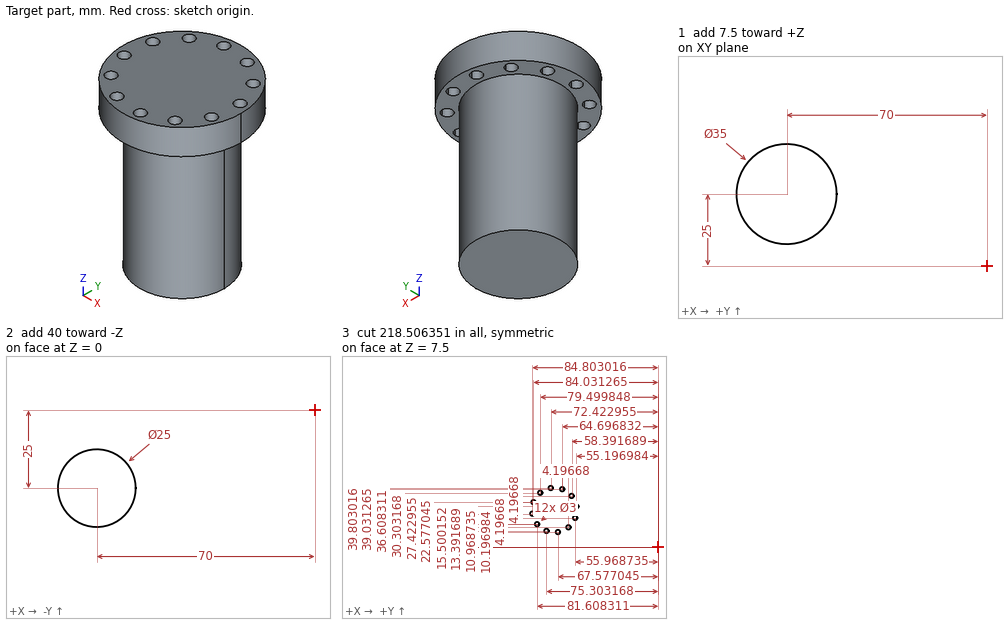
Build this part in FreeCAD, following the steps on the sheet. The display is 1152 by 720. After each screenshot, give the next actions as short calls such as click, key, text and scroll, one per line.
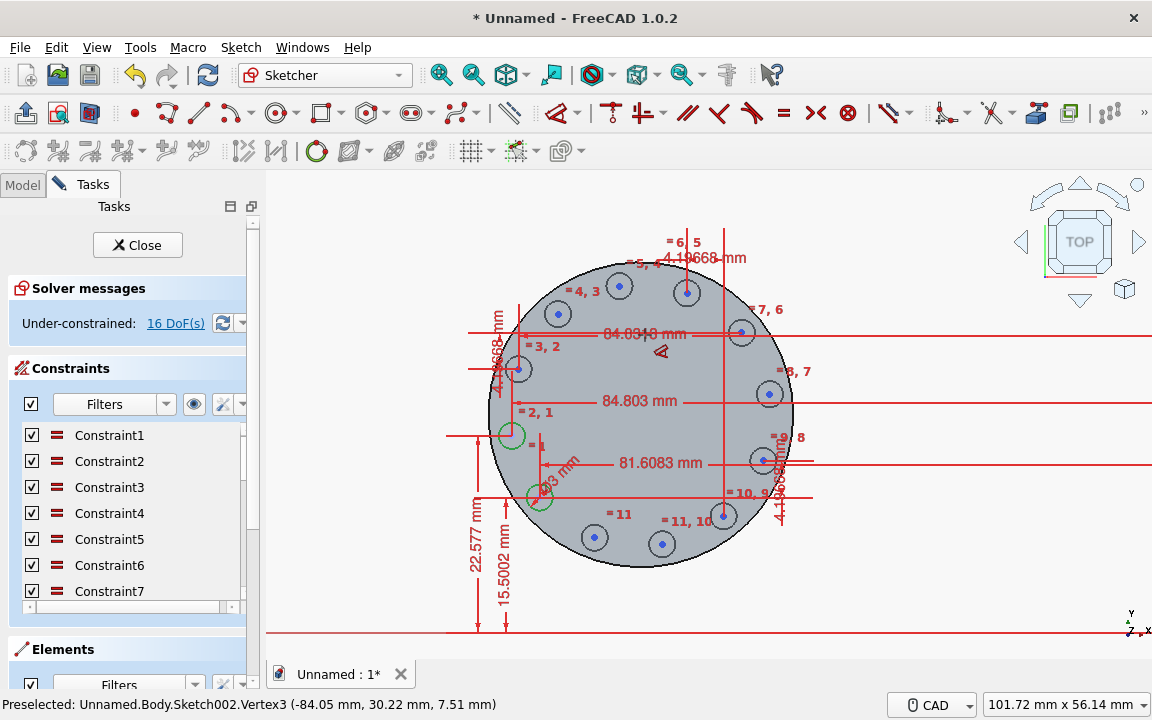
click(519, 369)
click(485, 500)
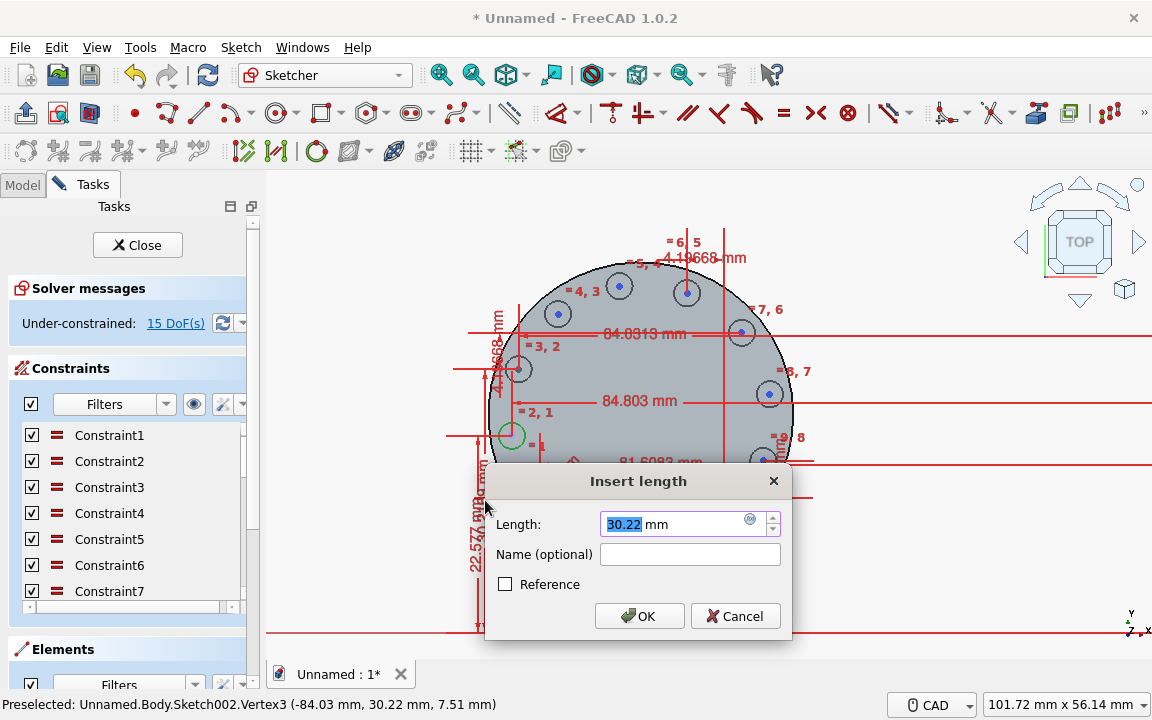
text(30.303168)
key(Return)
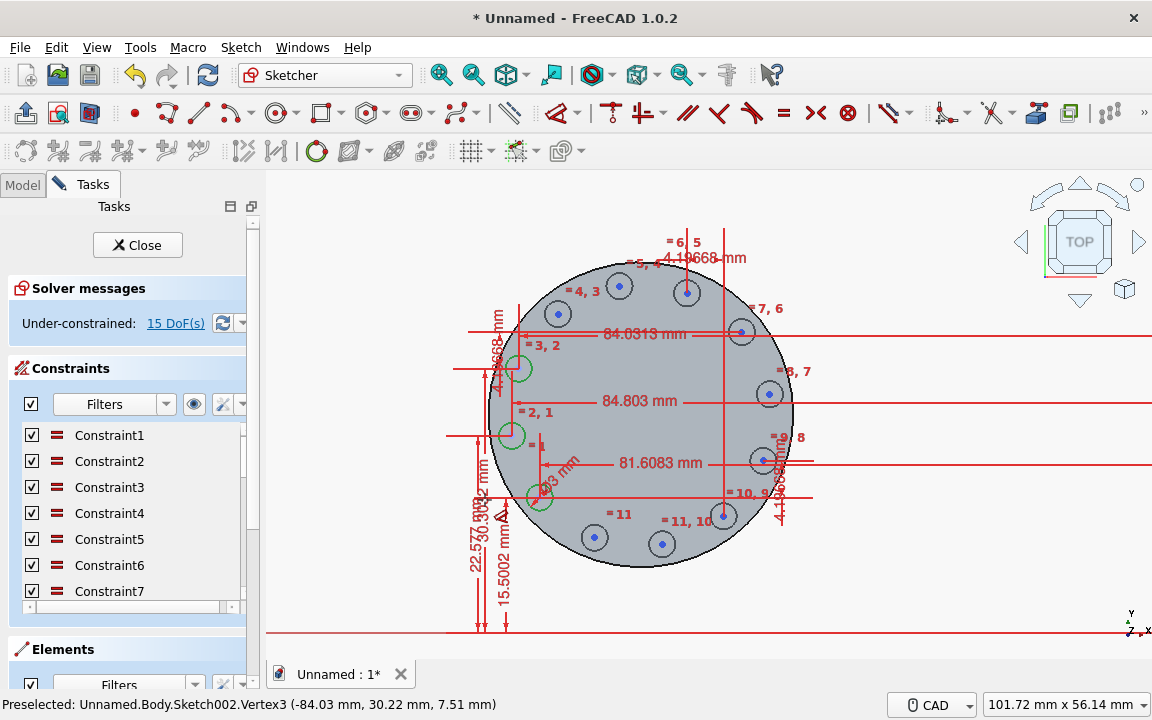
click(558, 314)
click(773, 280)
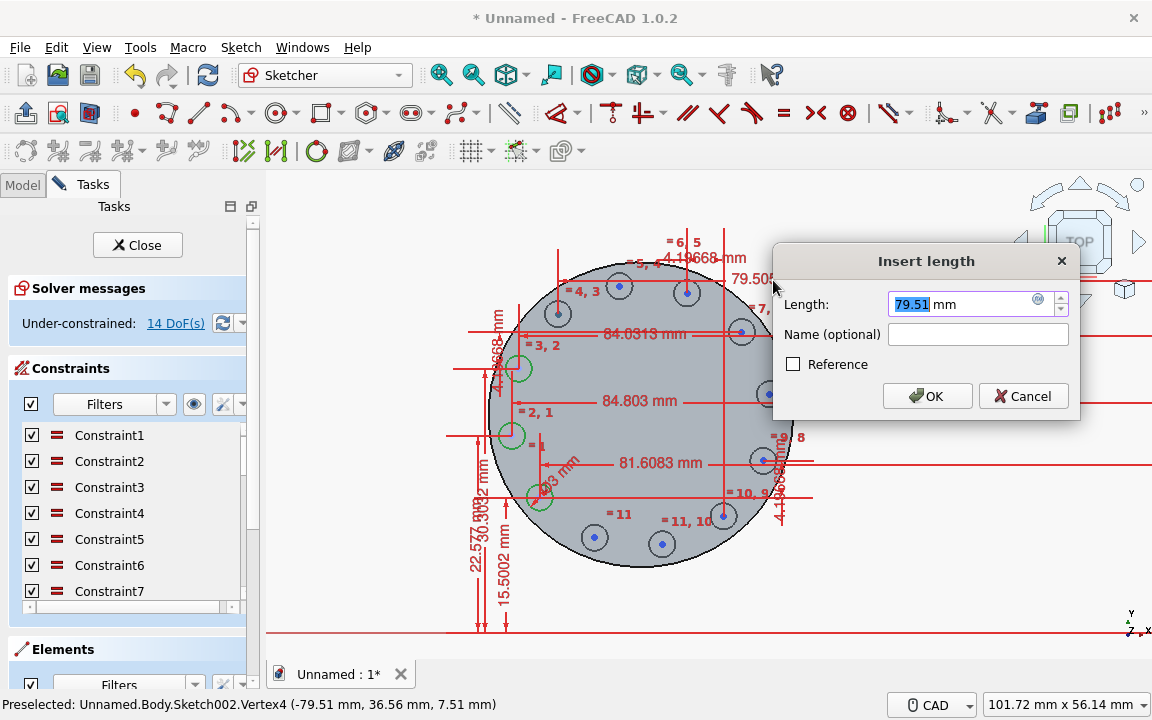
text(79.499848)
key(Return)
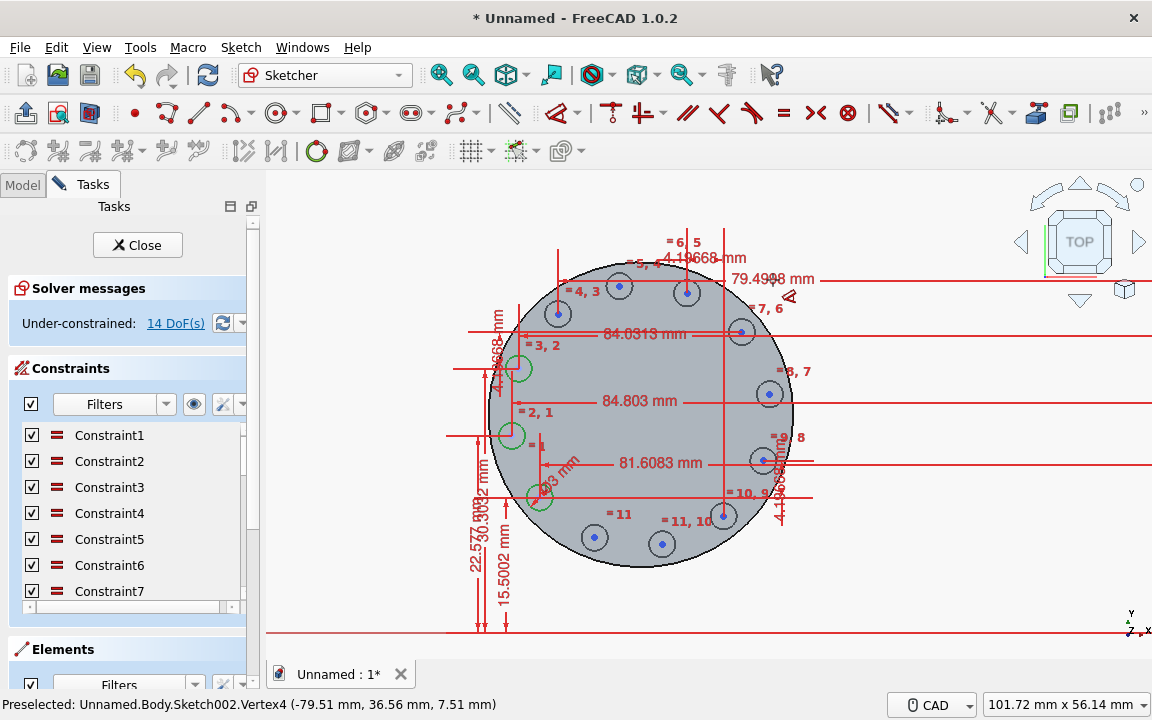
click(558, 314)
click(524, 400)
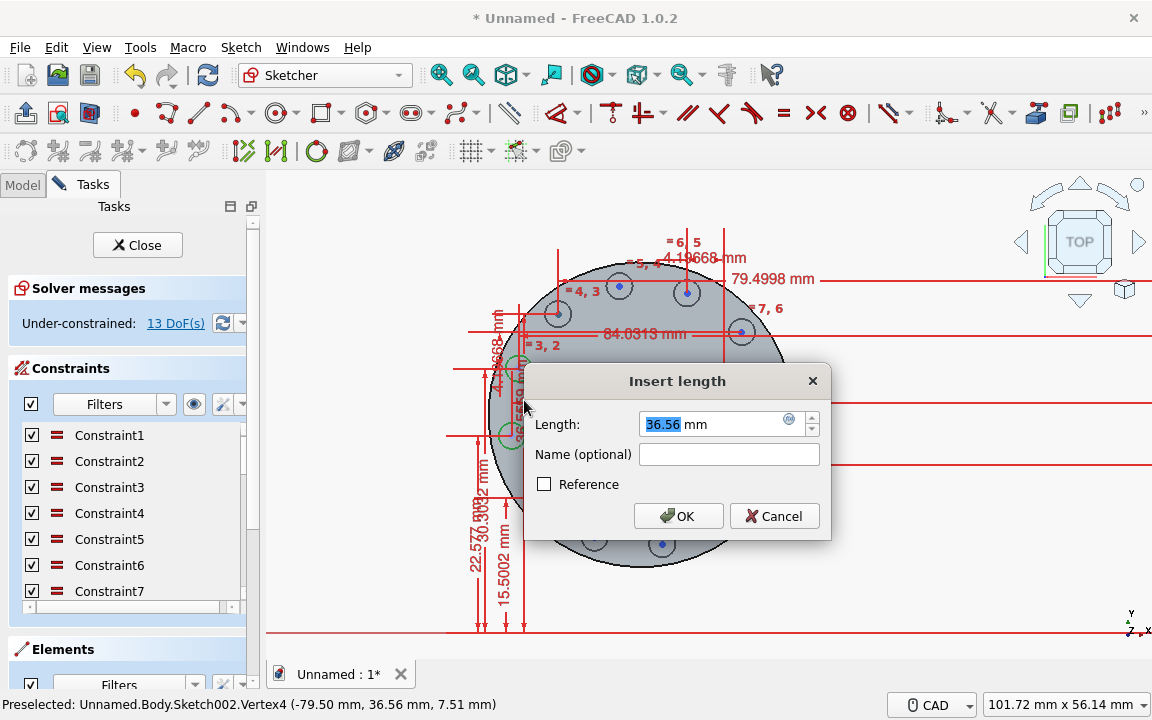
text(36.608311)
key(Return)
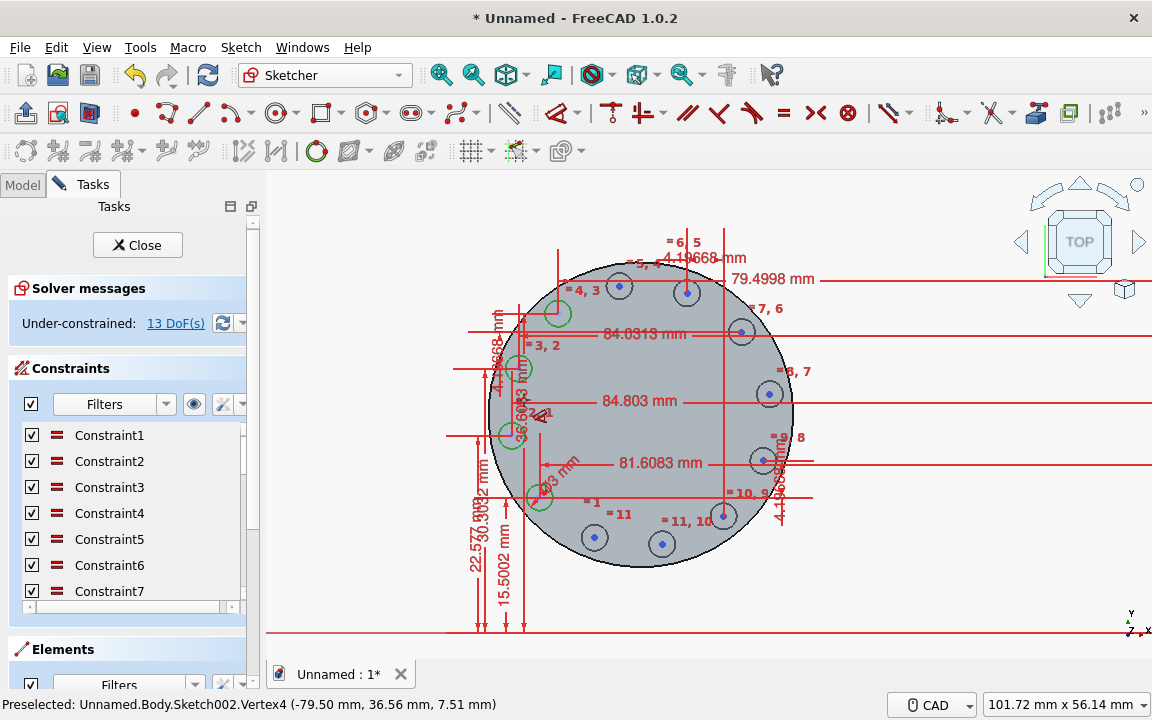
click(620, 286)
click(803, 252)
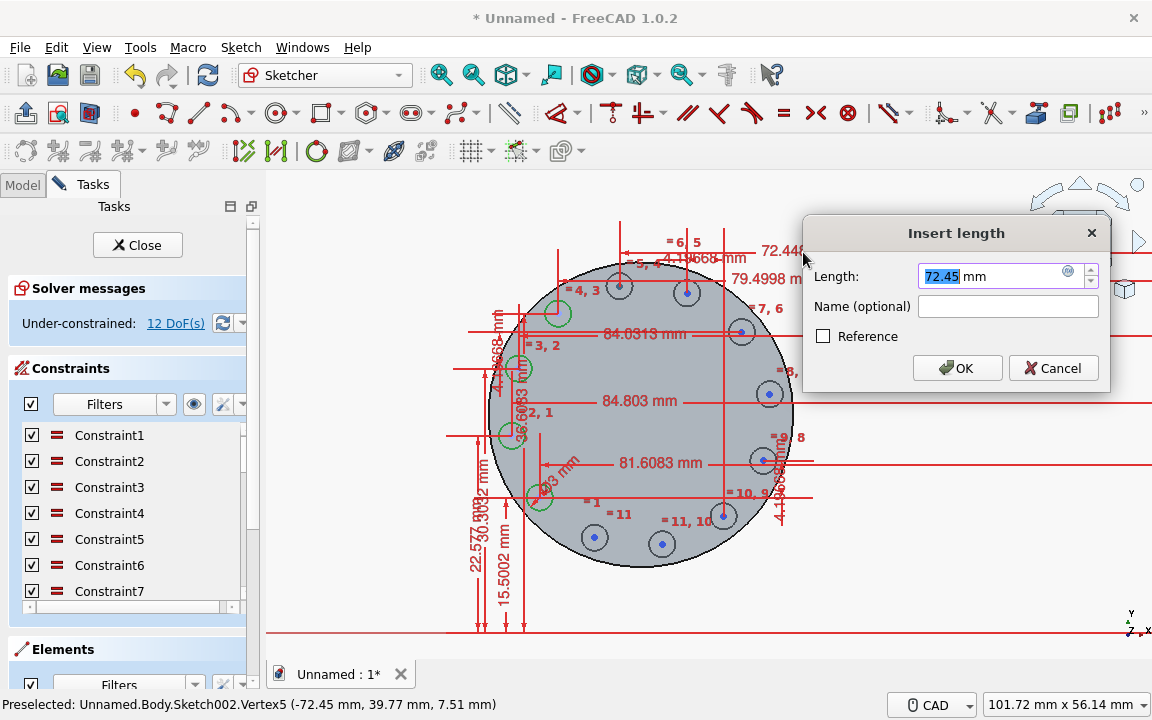
text(72.422955)
key(Return)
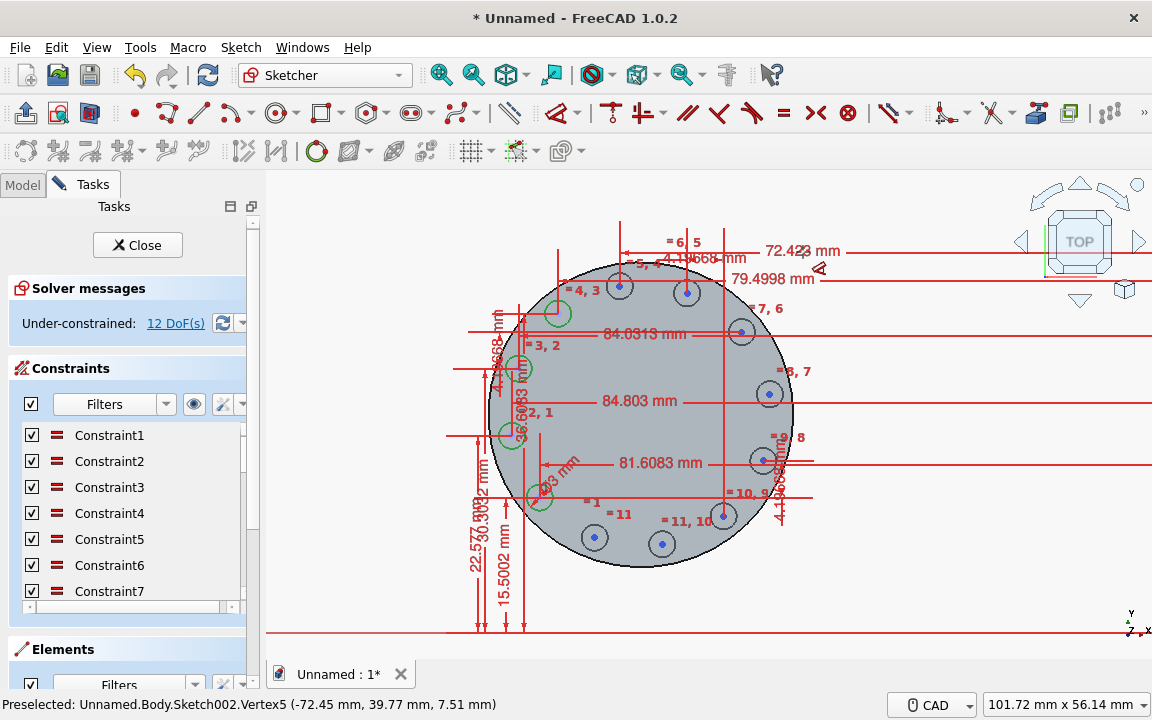
click(620, 286)
click(586, 379)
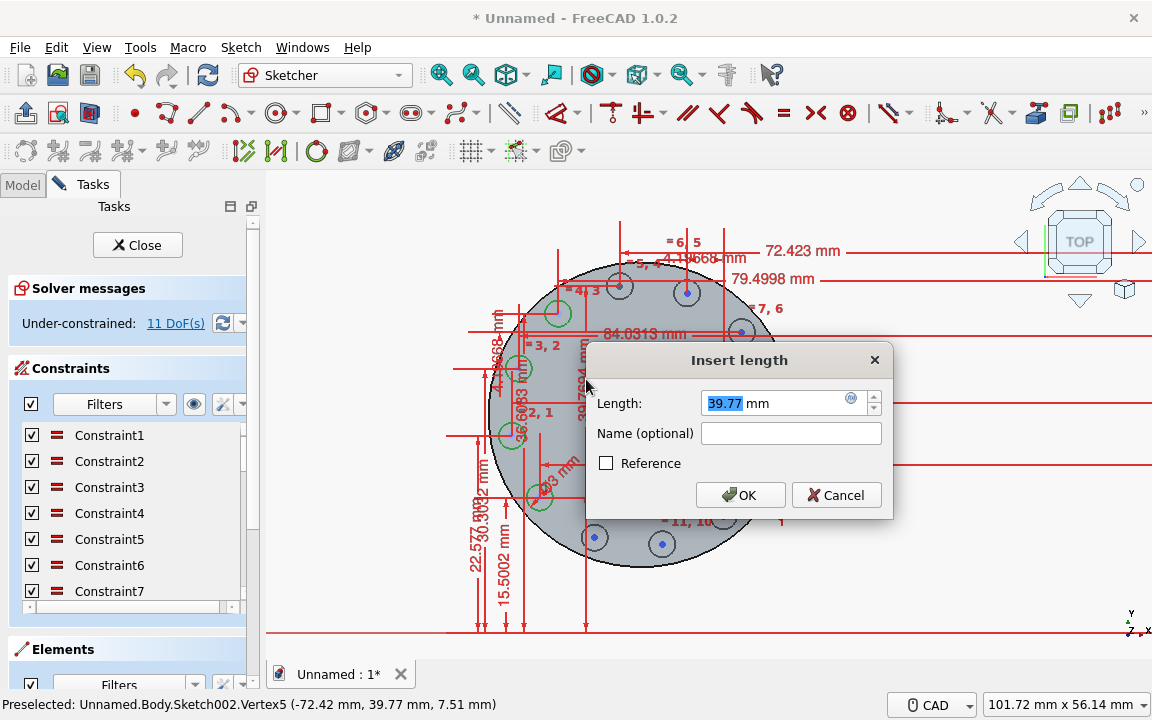
text(39.803016)
key(Return)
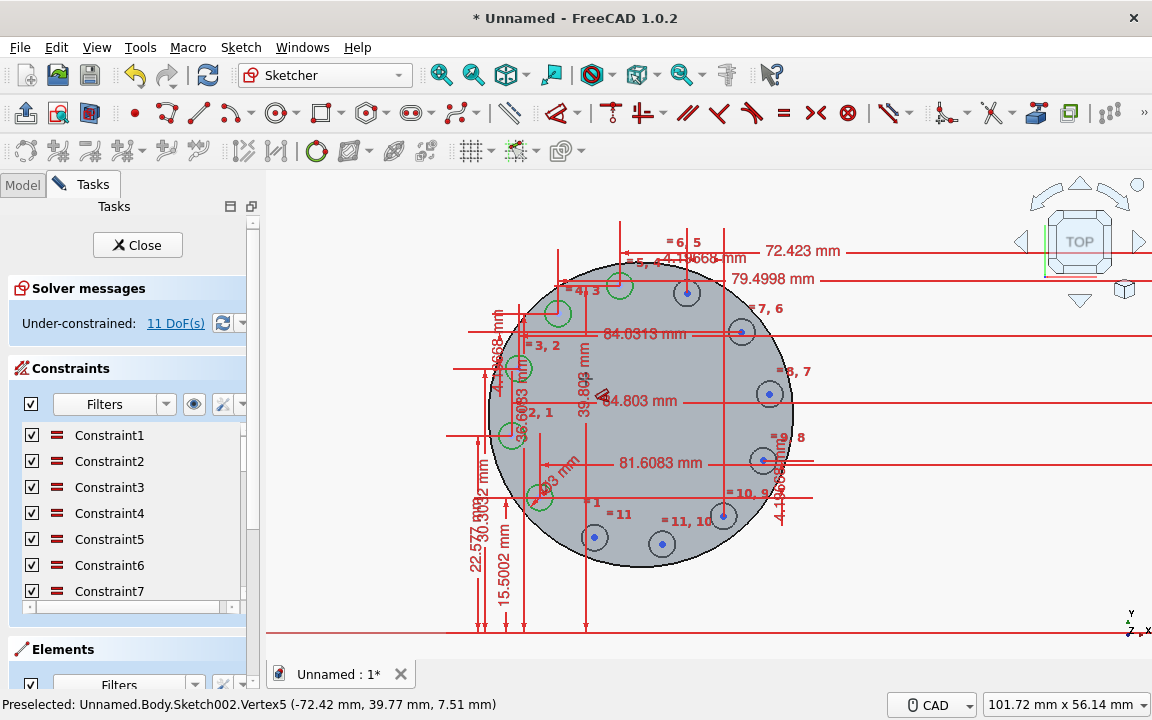
click(687, 293)
click(906, 259)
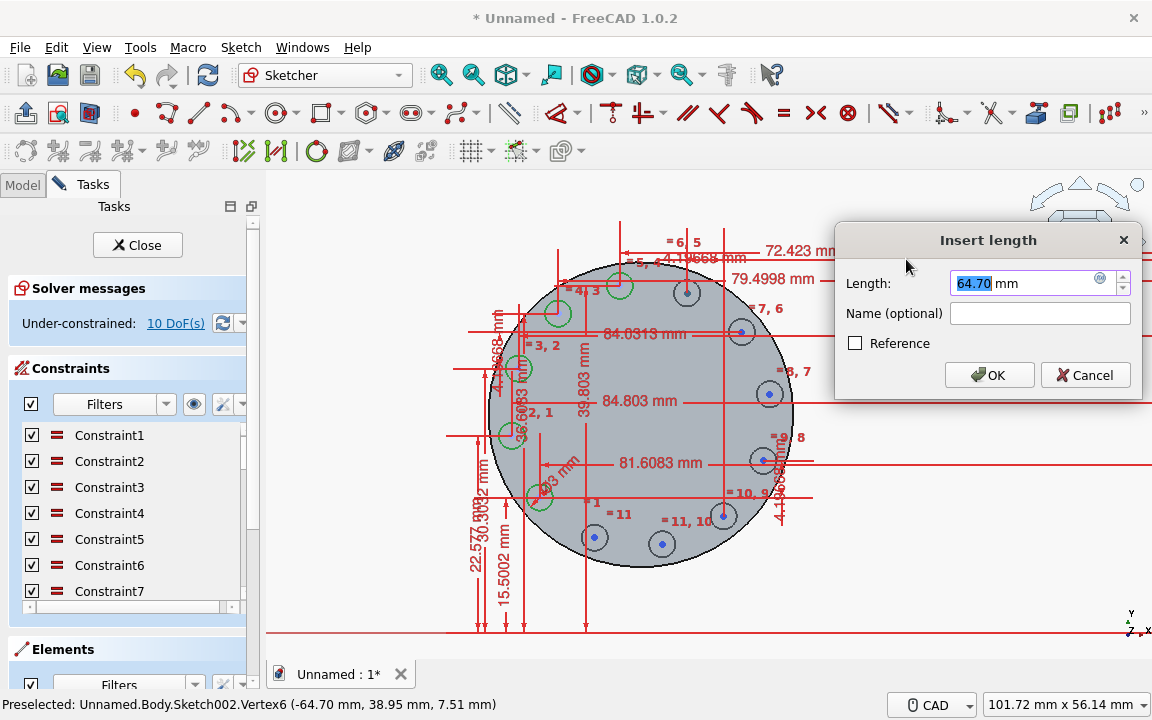
text(64.696832)
key(Return)